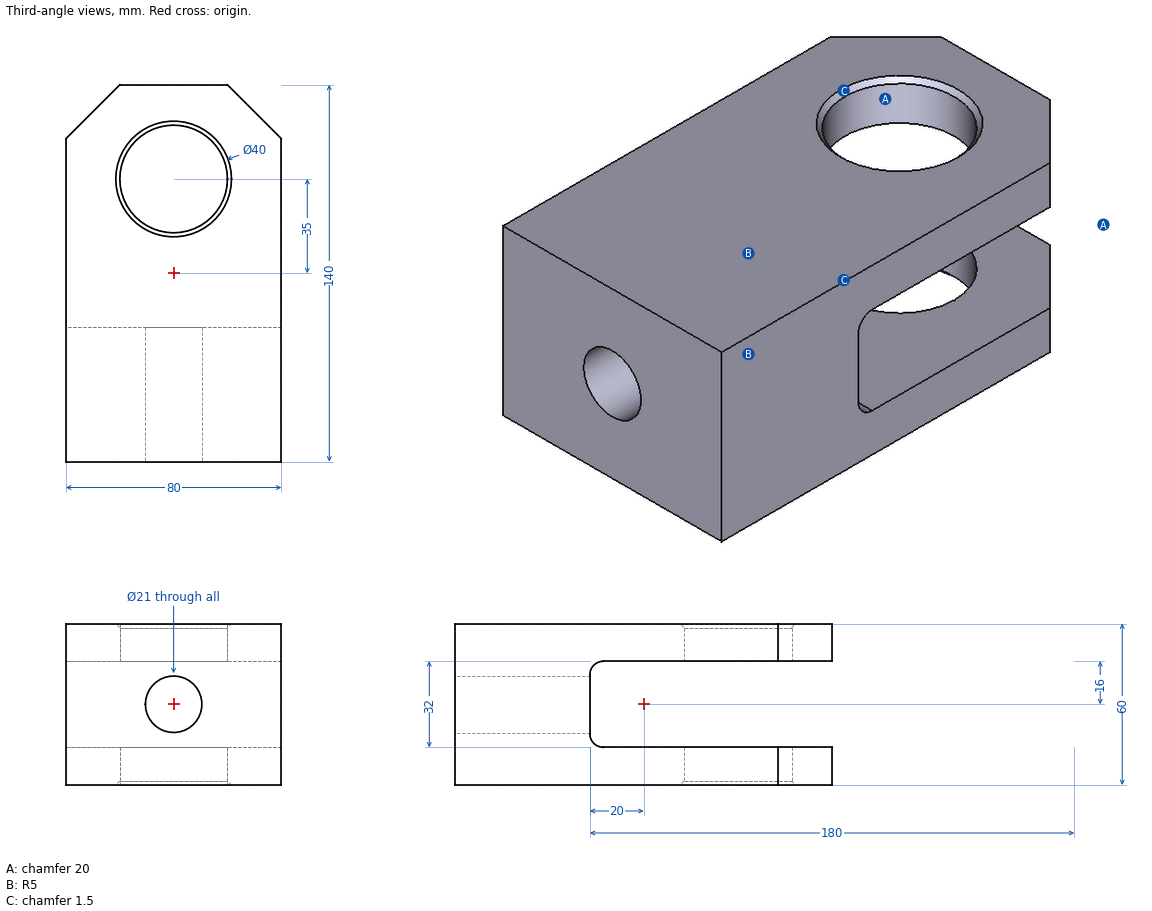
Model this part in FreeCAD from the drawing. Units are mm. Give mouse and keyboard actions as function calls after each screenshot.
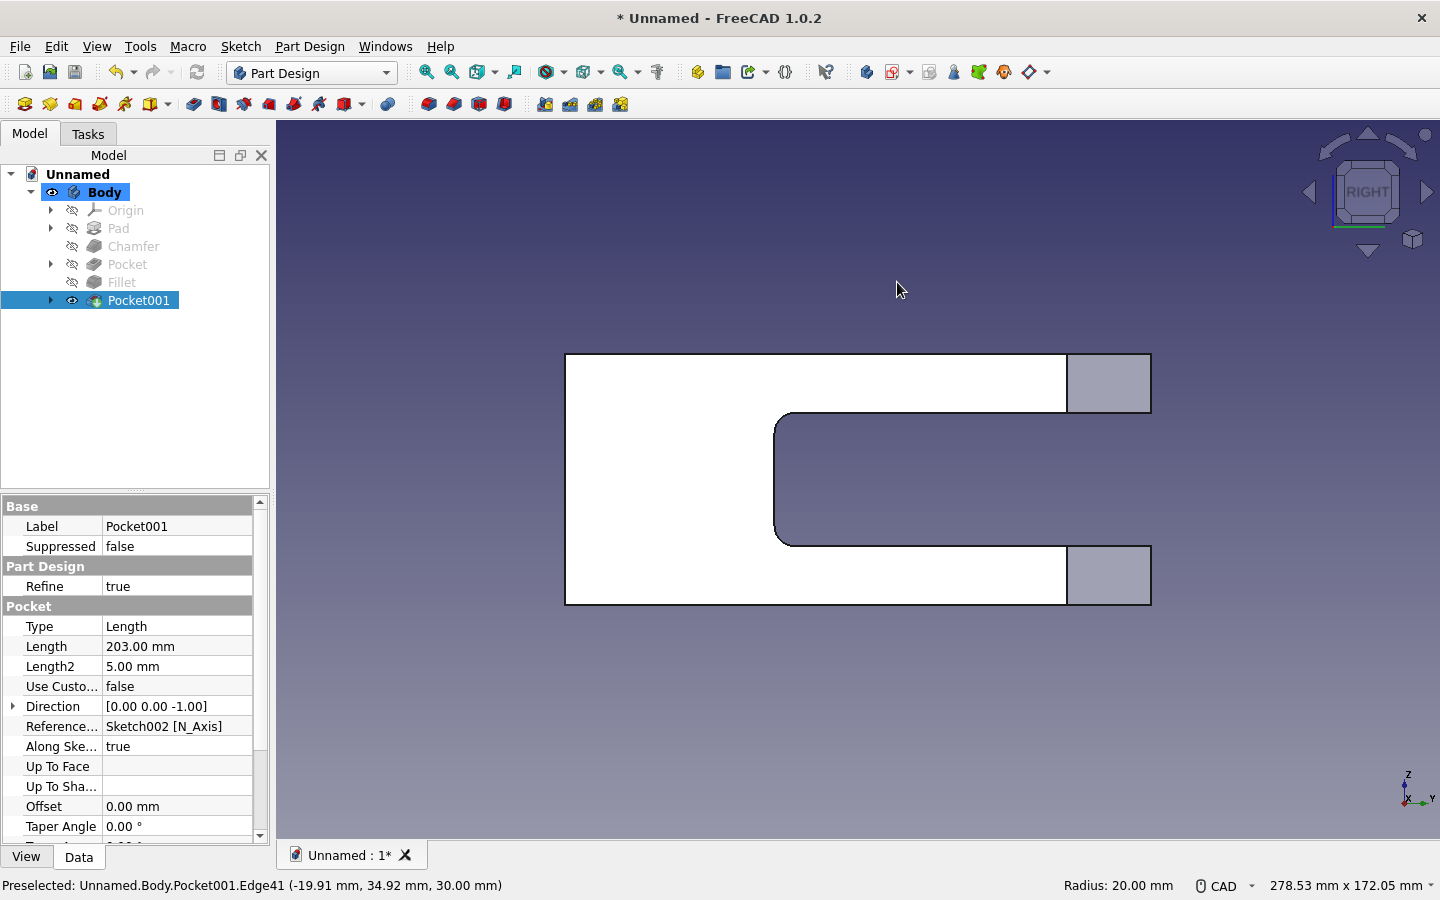
key(5)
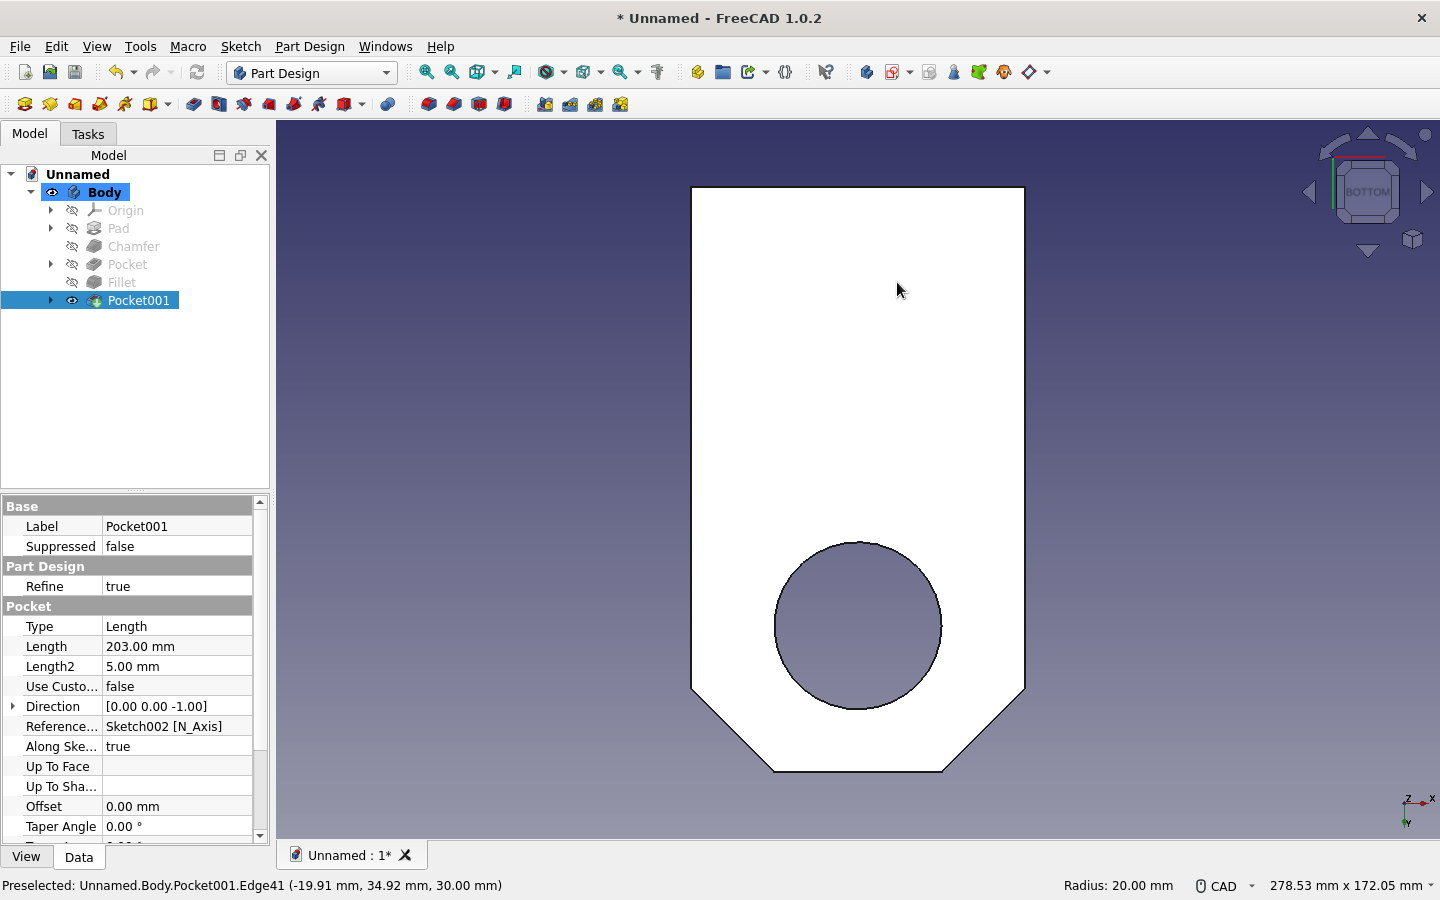
click(774, 625, ctrl)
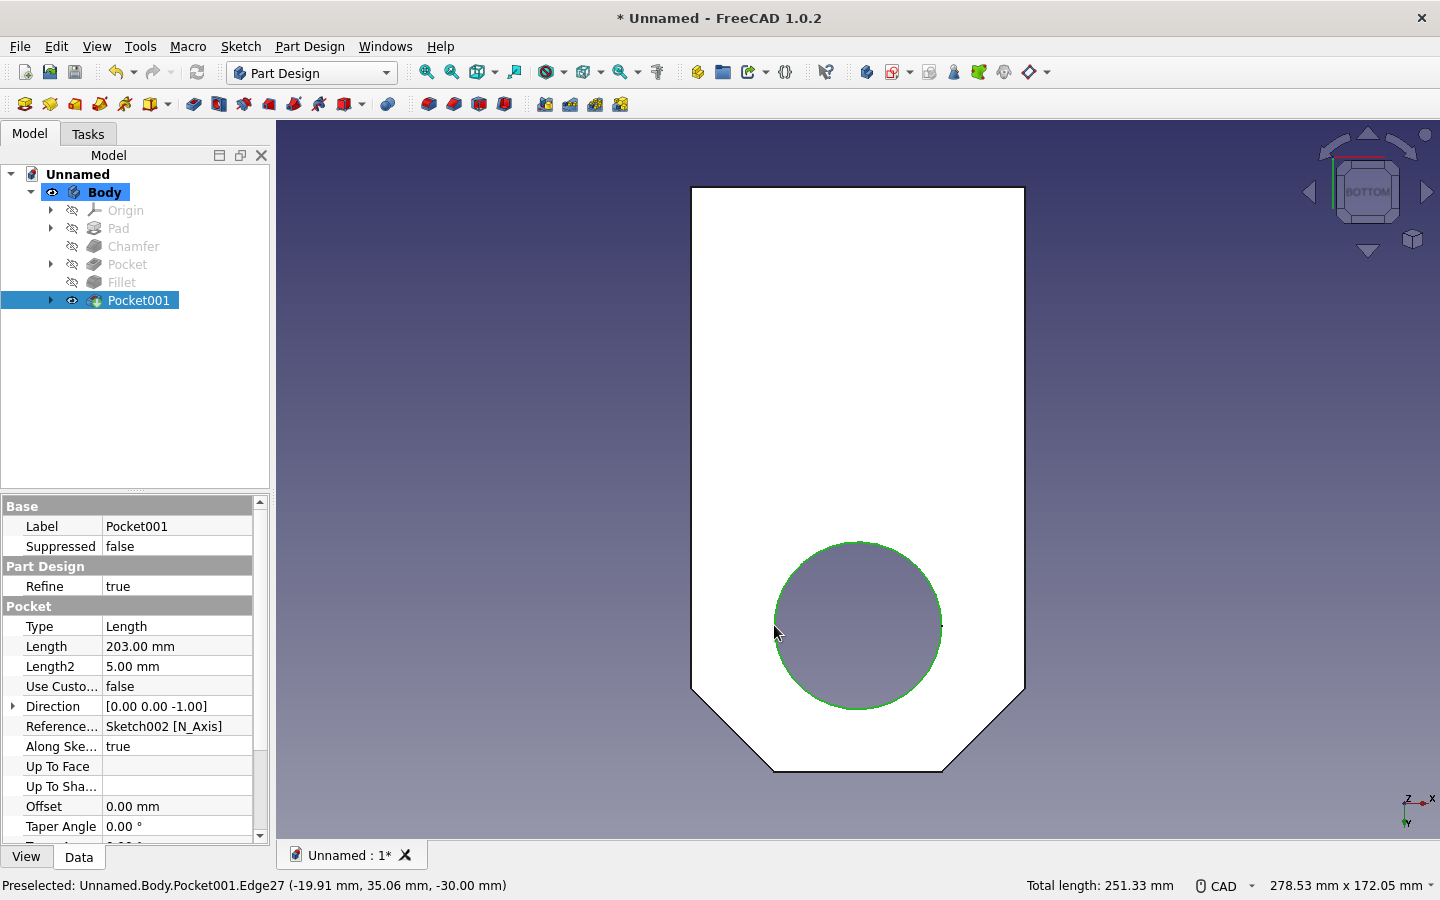
click(454, 104)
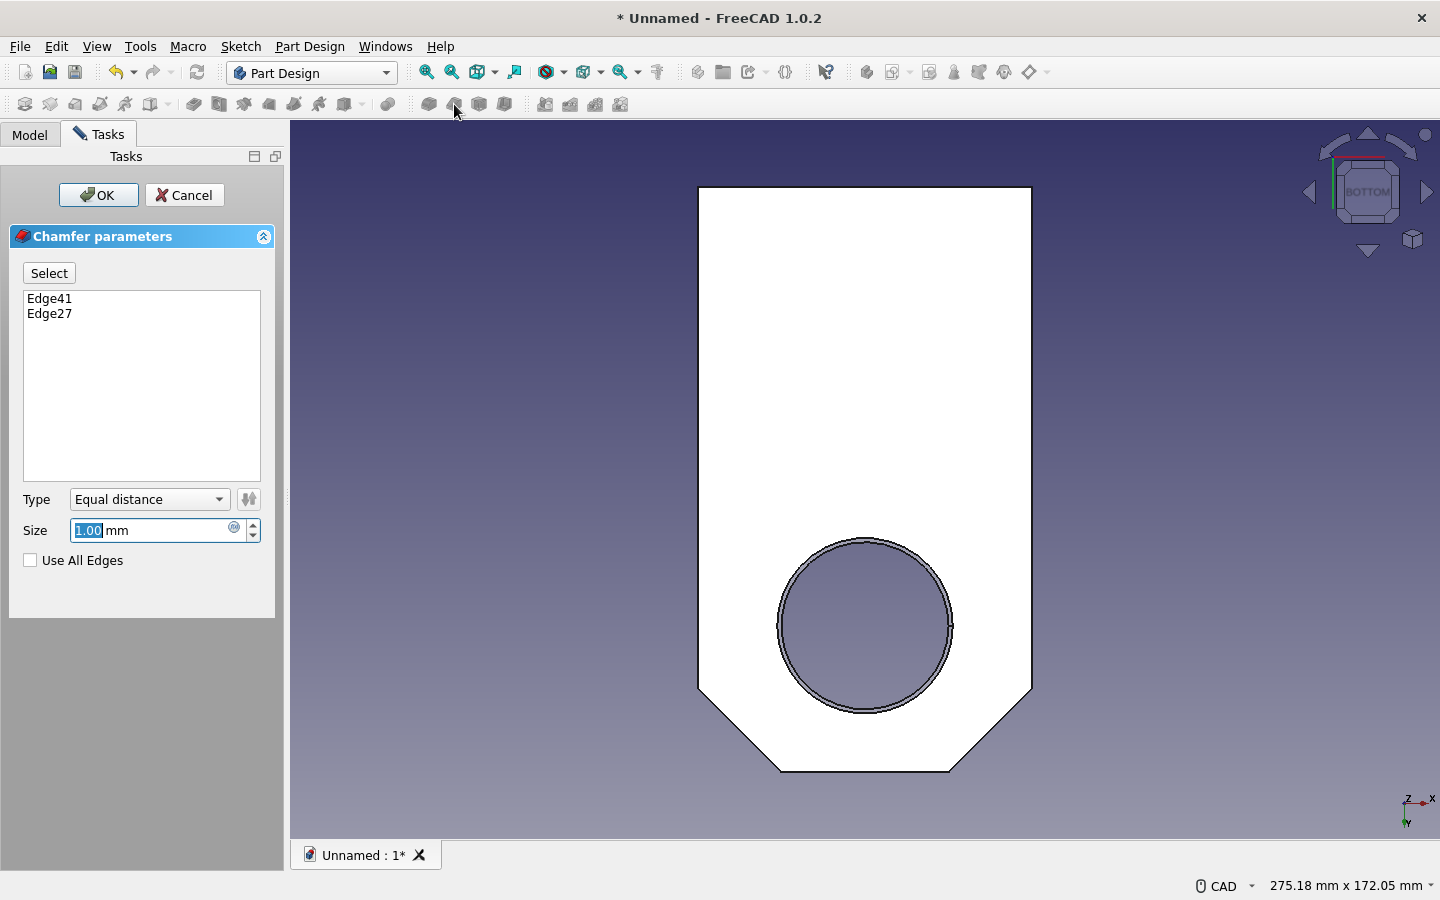
text(1.5)
key(Tab)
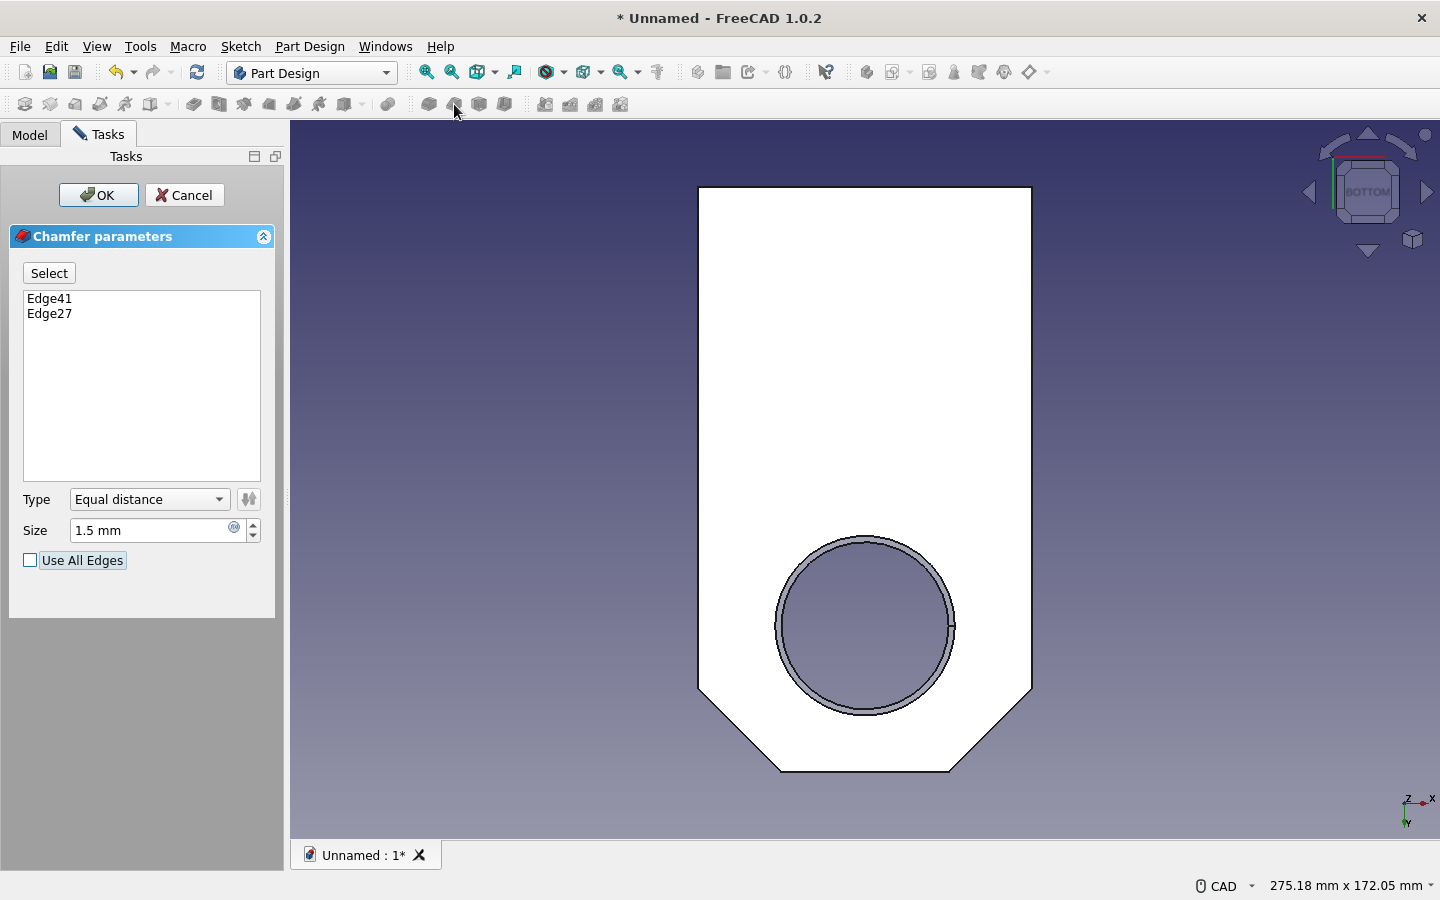
click(99, 195)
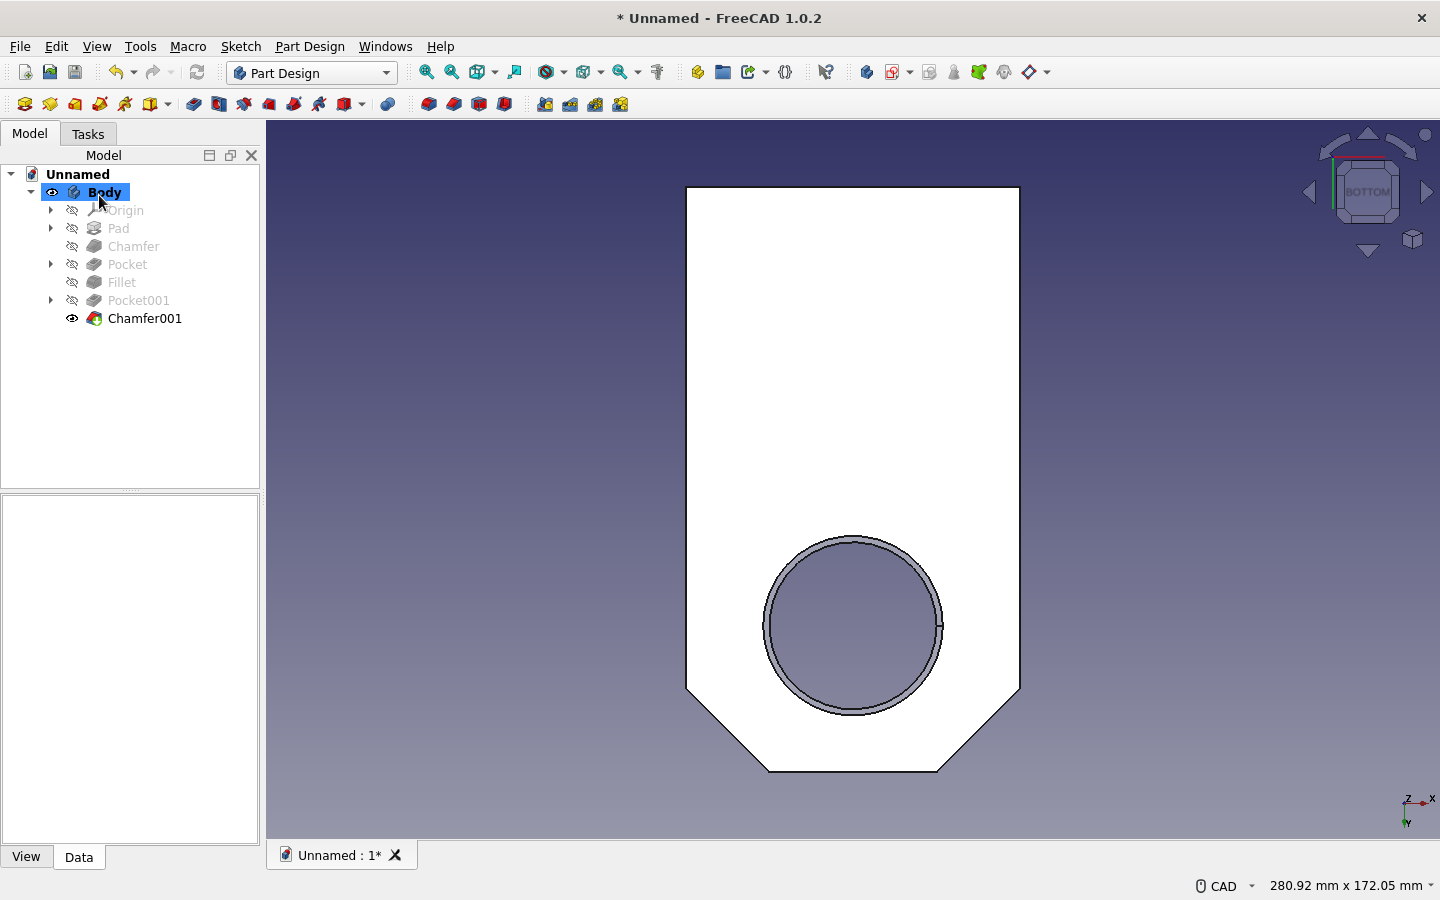
key(4)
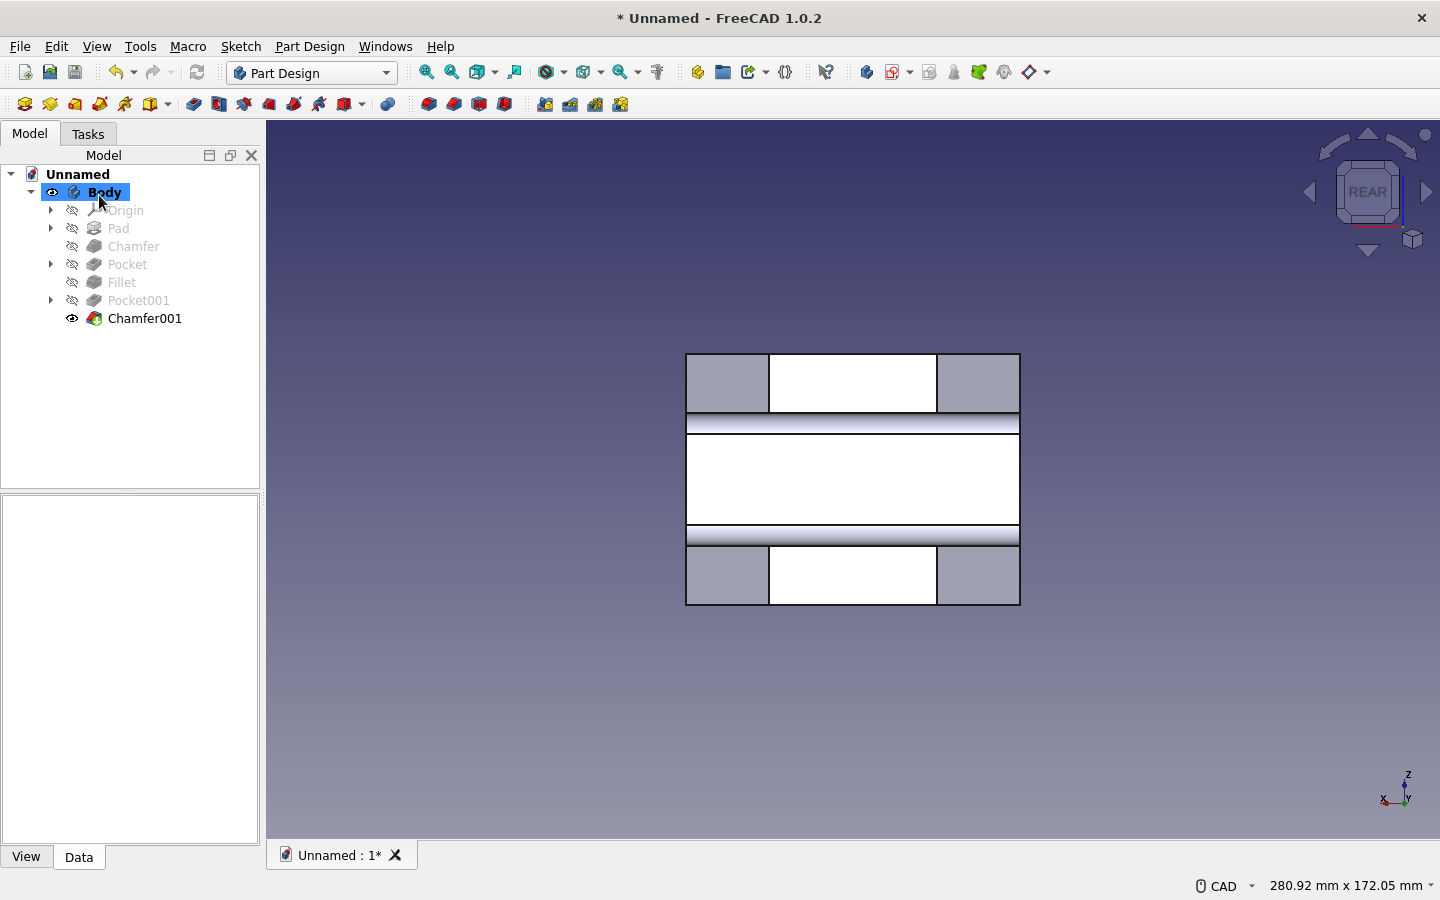
click(427, 72)